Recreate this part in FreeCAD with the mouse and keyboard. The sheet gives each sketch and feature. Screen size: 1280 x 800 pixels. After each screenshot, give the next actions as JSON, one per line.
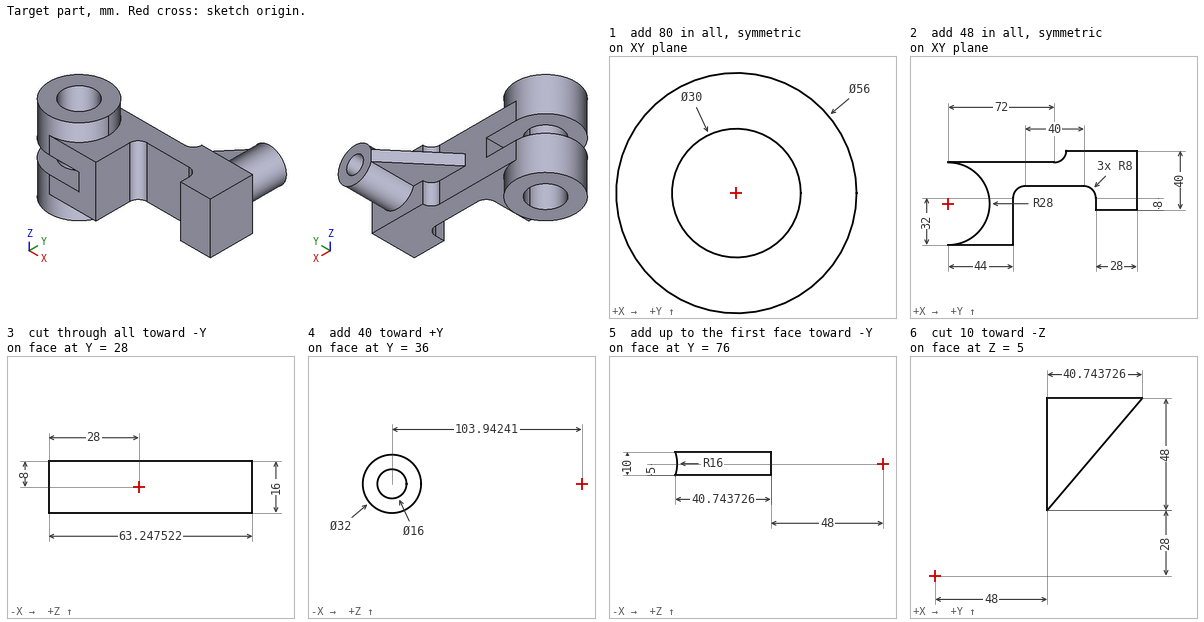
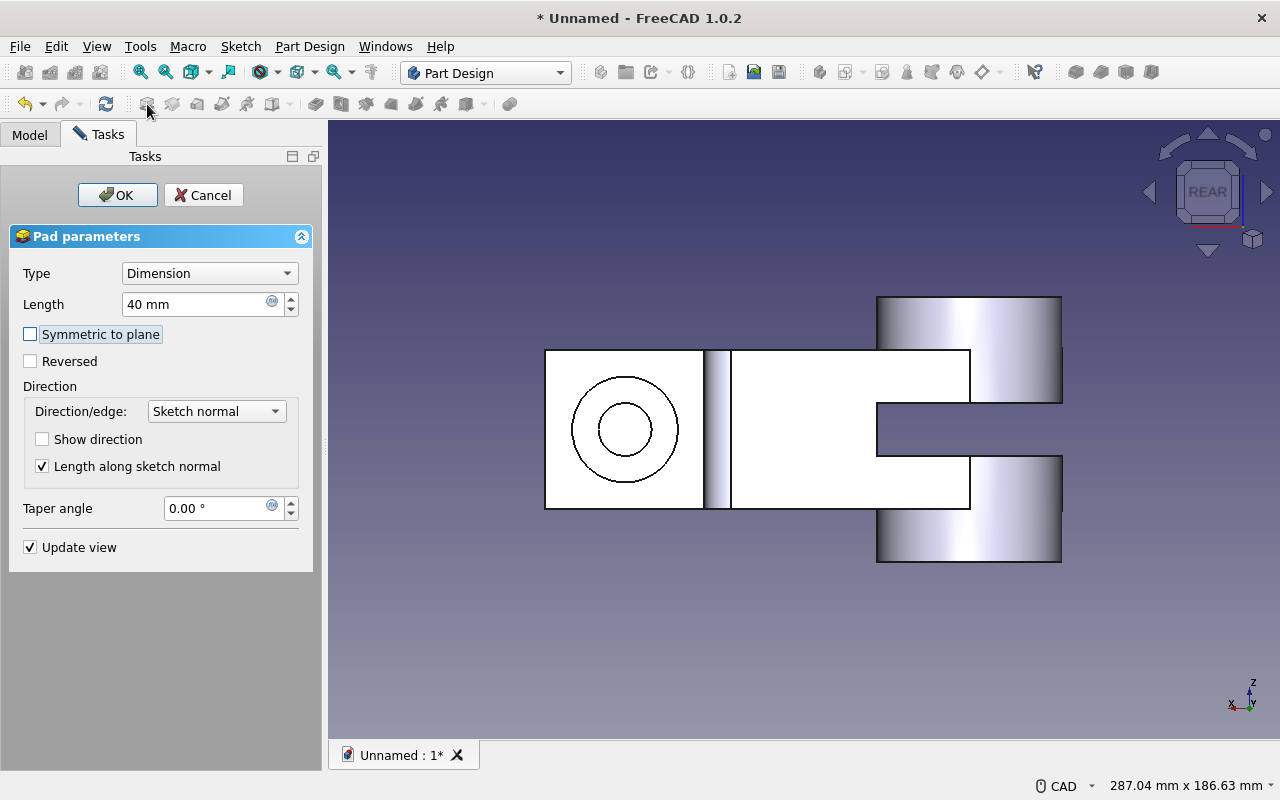
{"action": "left_click", "coordinate": [118, 195]}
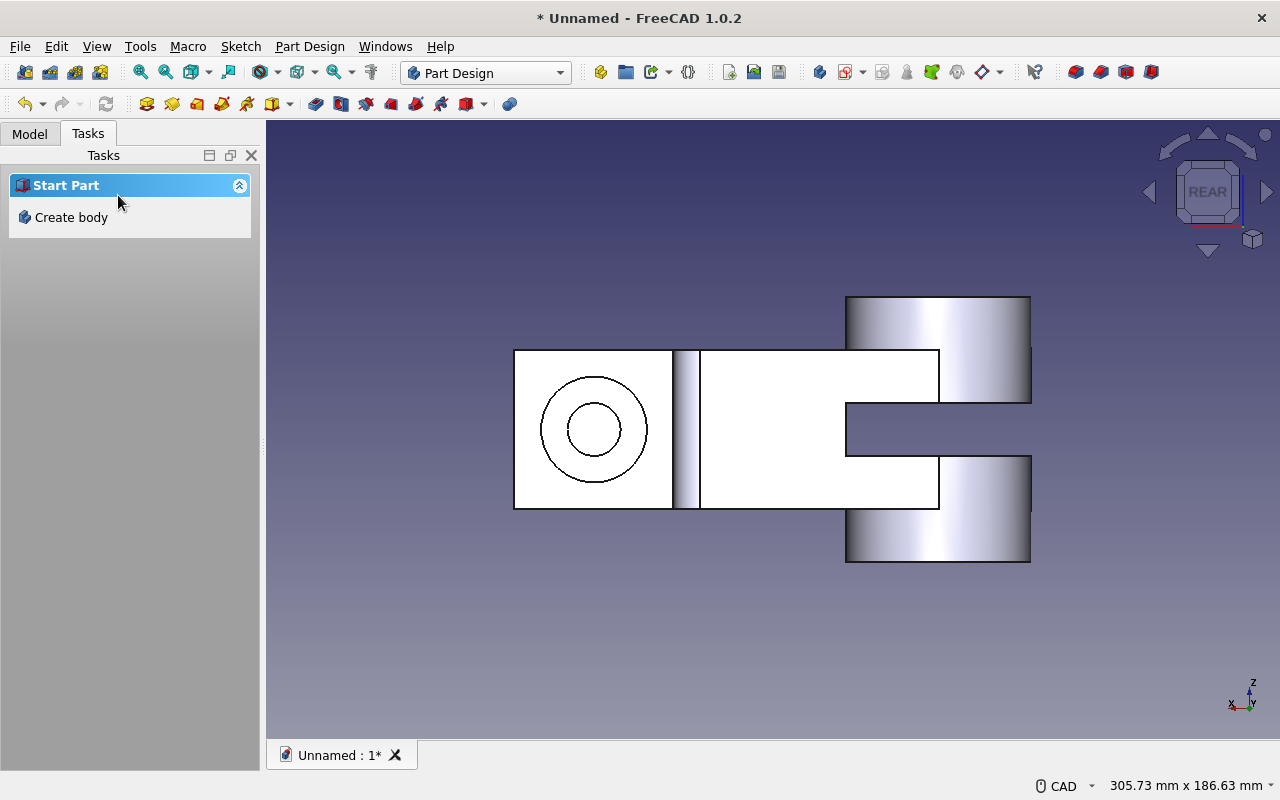
{"action": "left_click", "coordinate": [564, 459]}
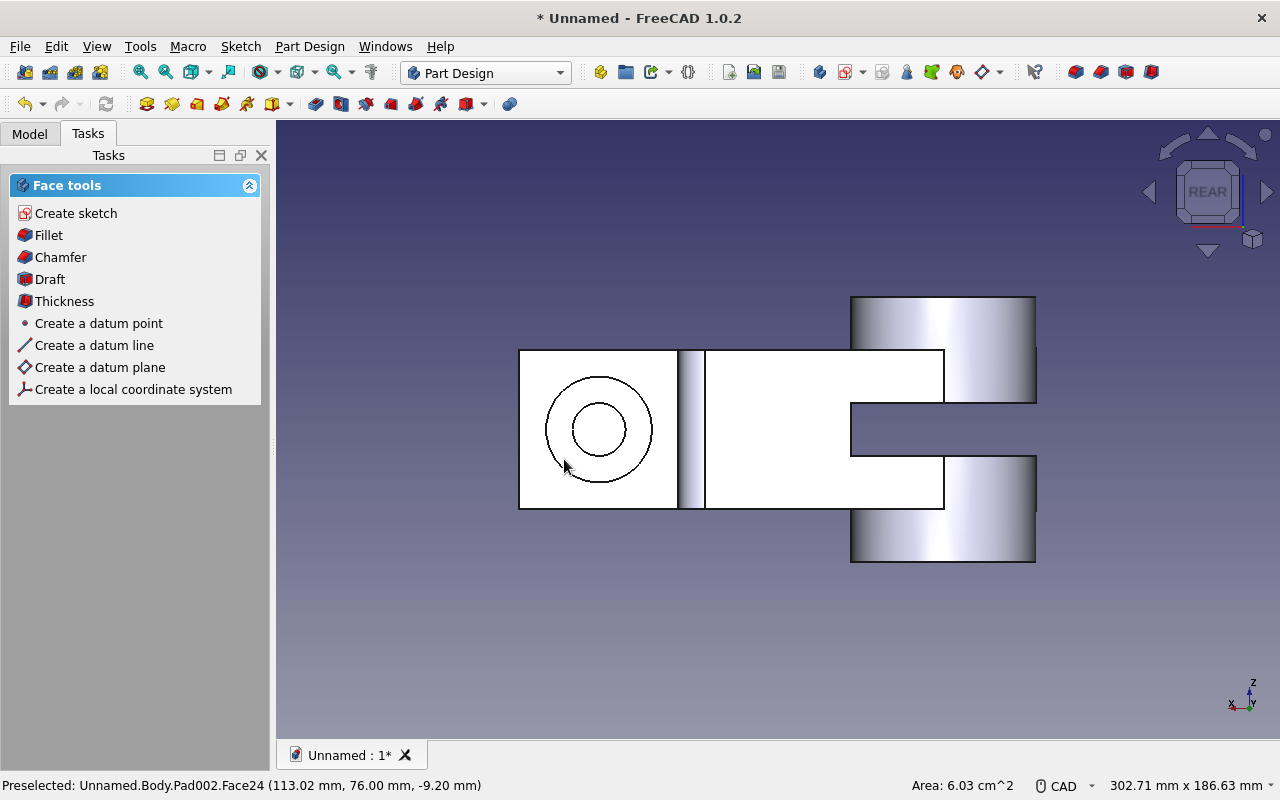
{"action": "left_click", "coordinate": [844, 72]}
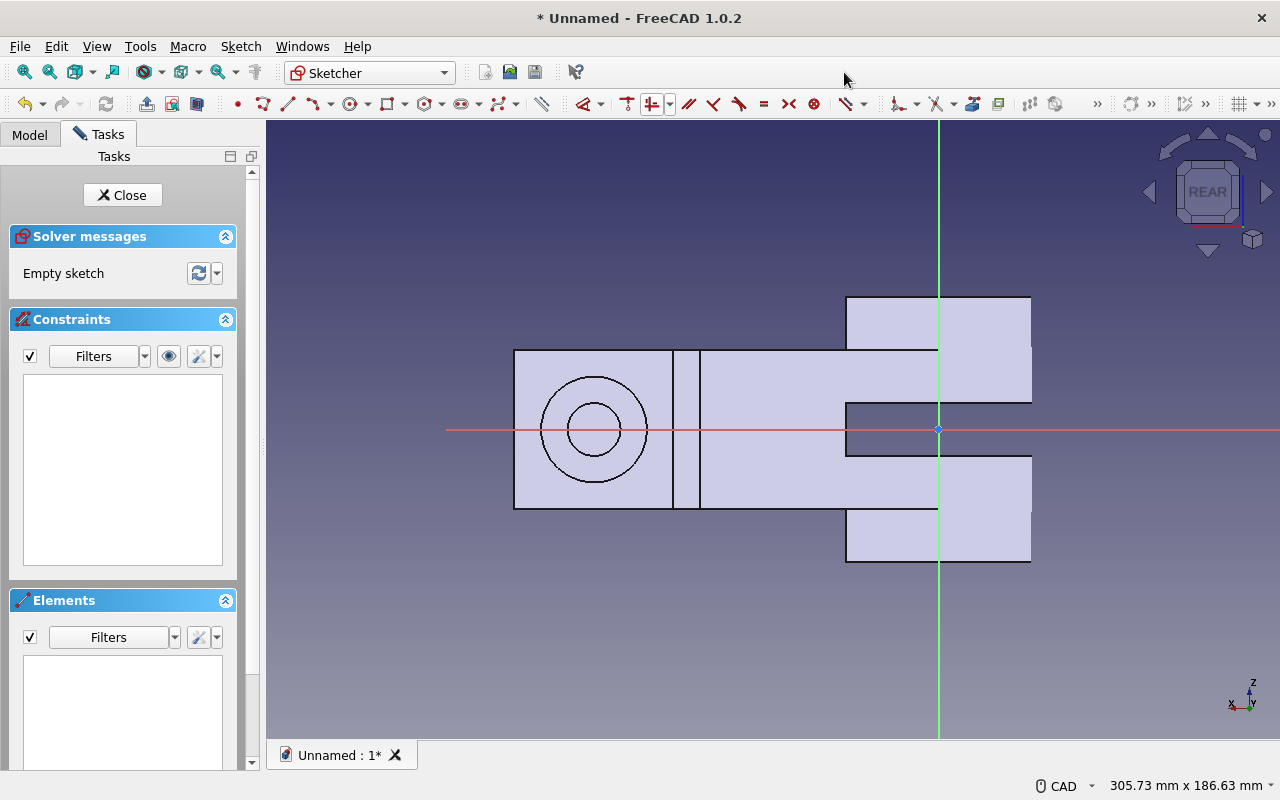
{"action": "scroll", "coordinate": [898, 430], "scroll_direction": "up", "scroll_amount": 3}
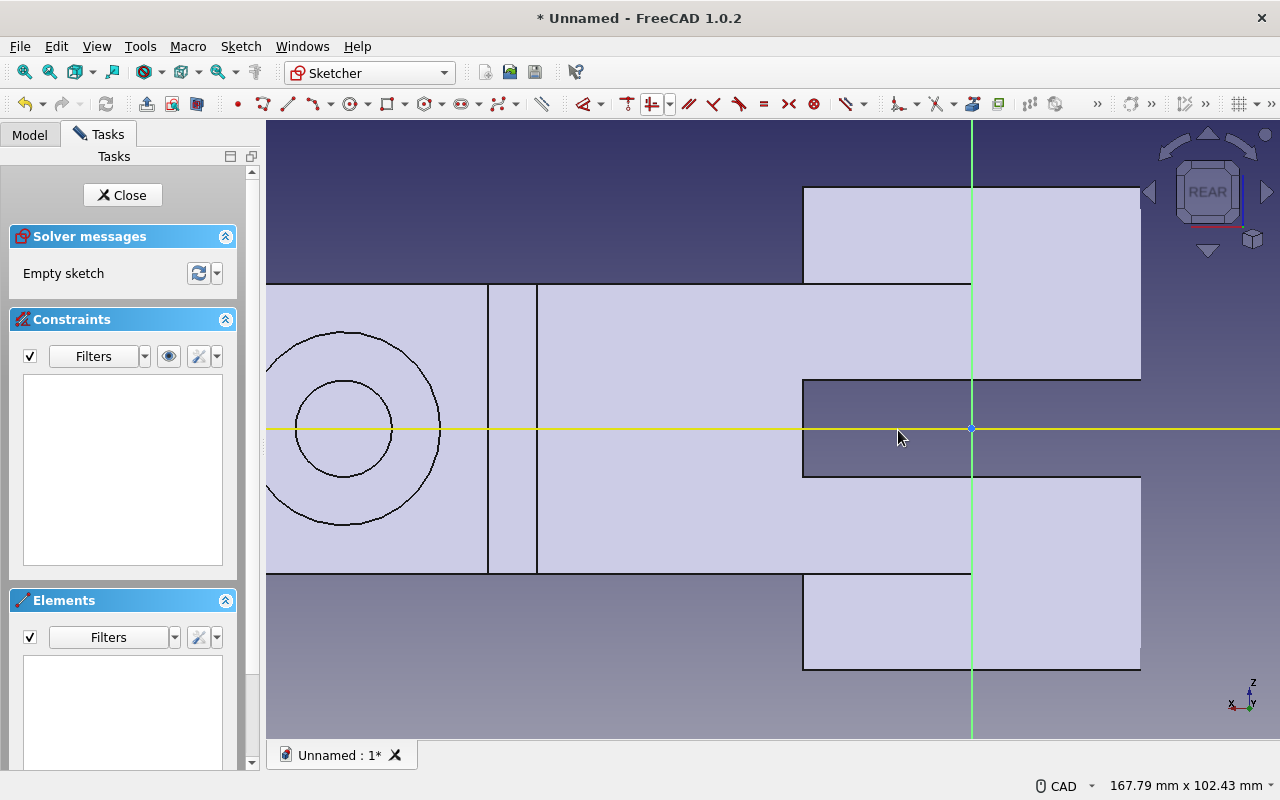
{"action": "left_click", "coordinate": [263, 104]}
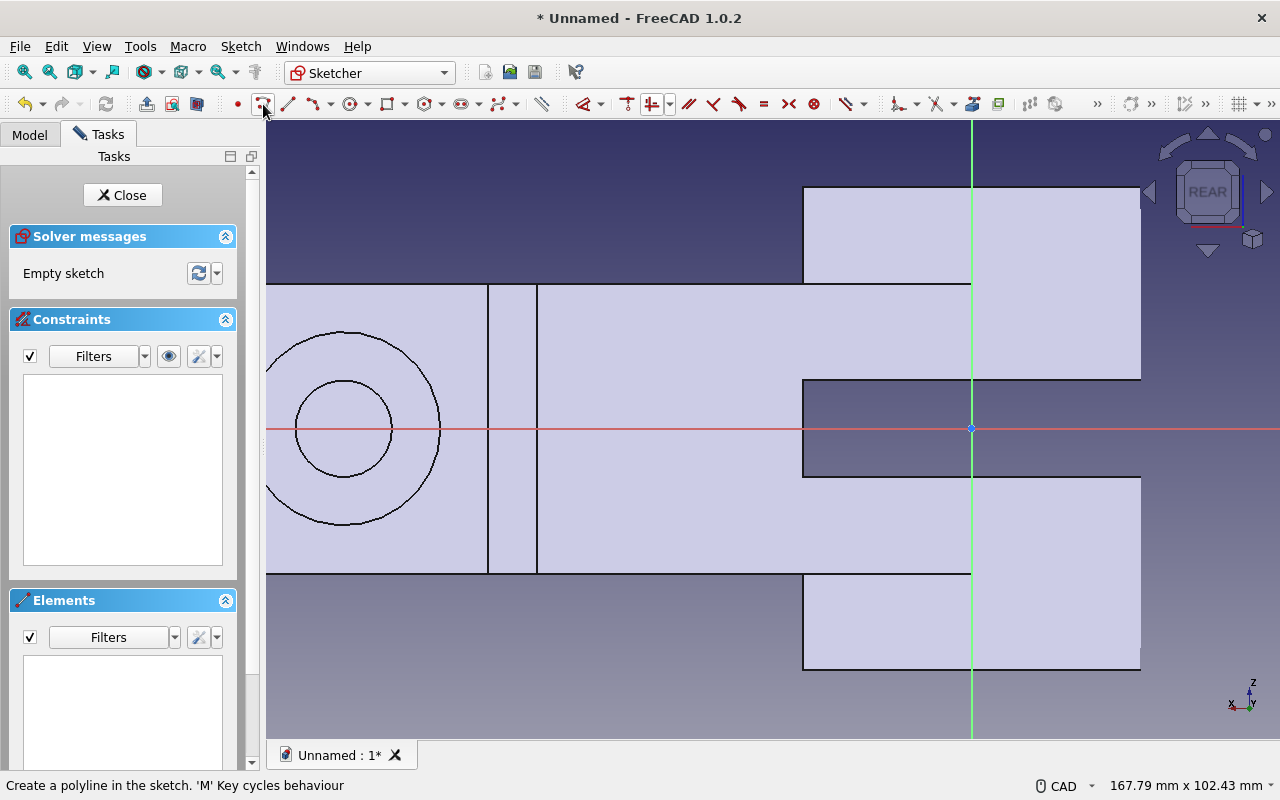
{"action": "left_click", "coordinate": [436, 459]}
{"action": "left_click", "coordinate": [682, 459]}
{"action": "left_click", "coordinate": [682, 398]}
{"action": "left_click", "coordinate": [436, 398]}
{"action": "right_click", "coordinate": [436, 398]}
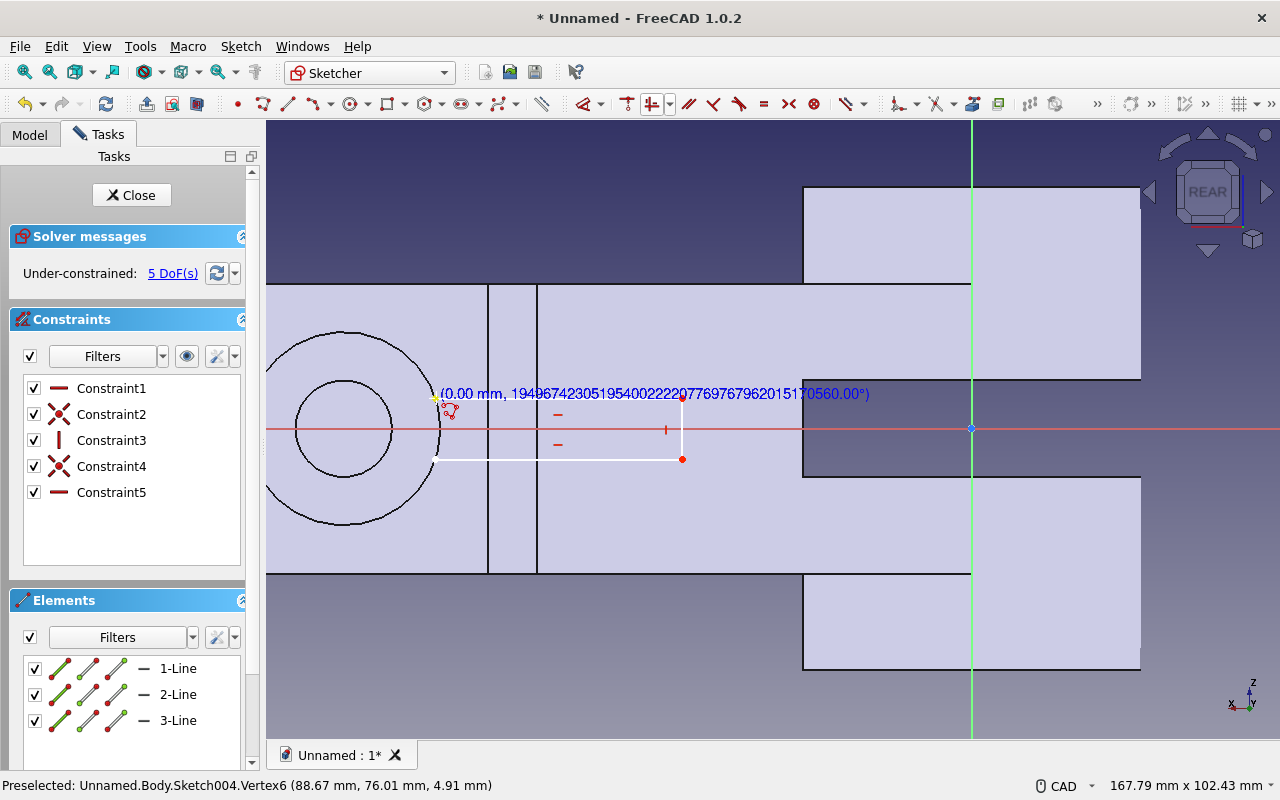
{"action": "left_click", "coordinate": [312, 104]}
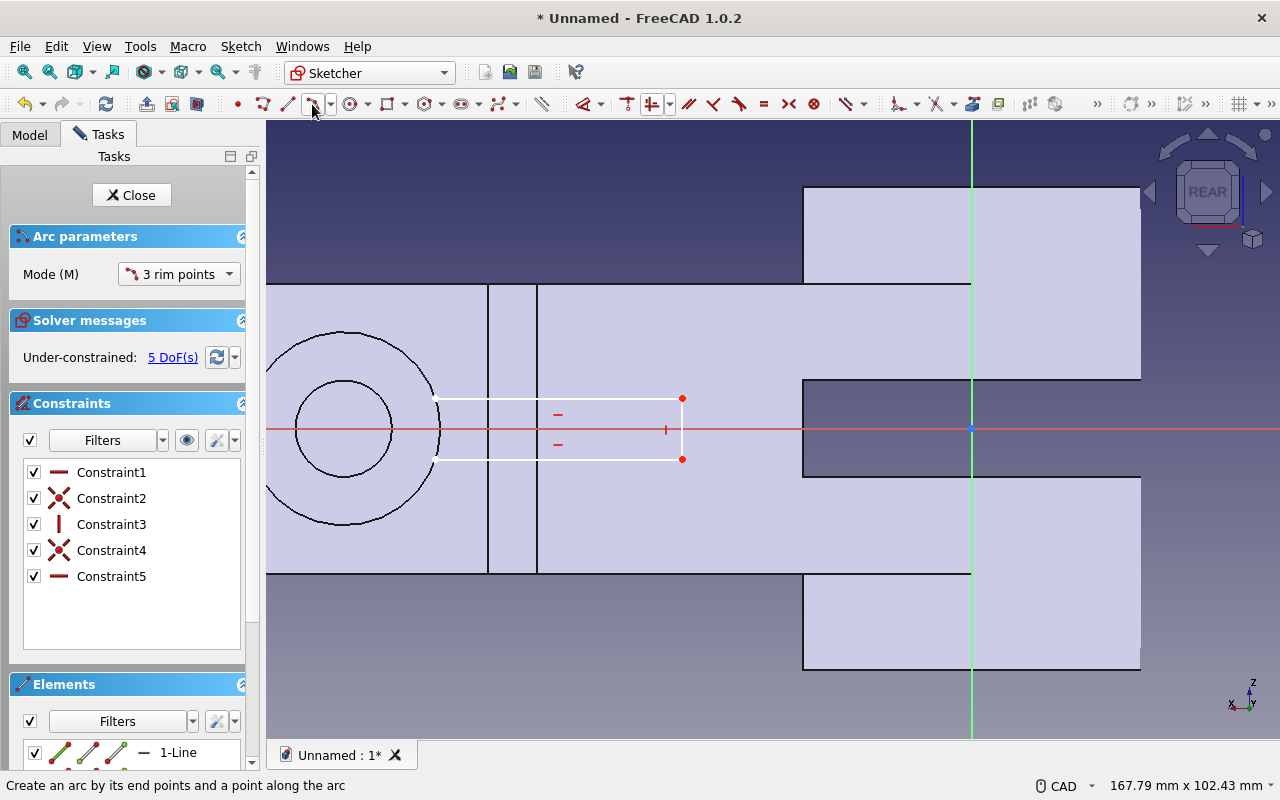
{"action": "left_click", "coordinate": [436, 399]}
{"action": "left_click", "coordinate": [436, 460]}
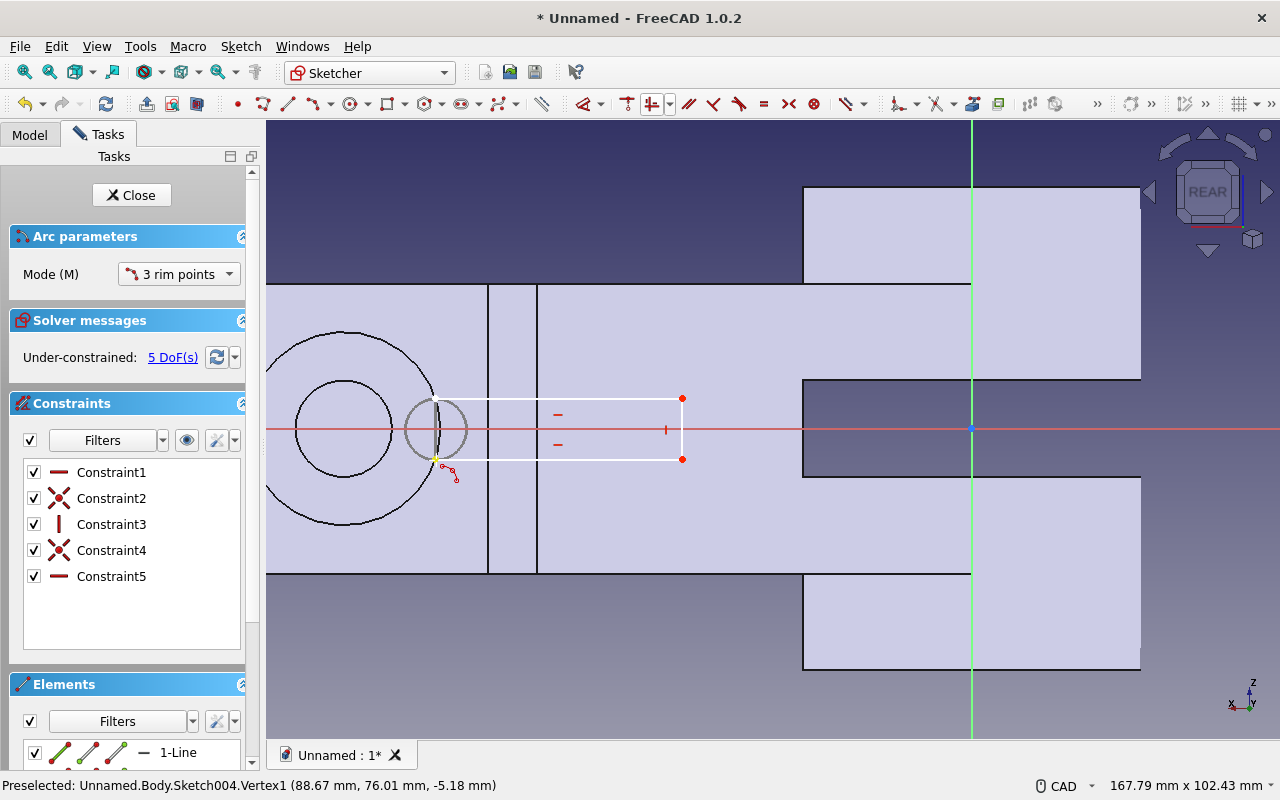
{"action": "scroll", "coordinate": [440, 435], "scroll_direction": "up", "scroll_amount": 7}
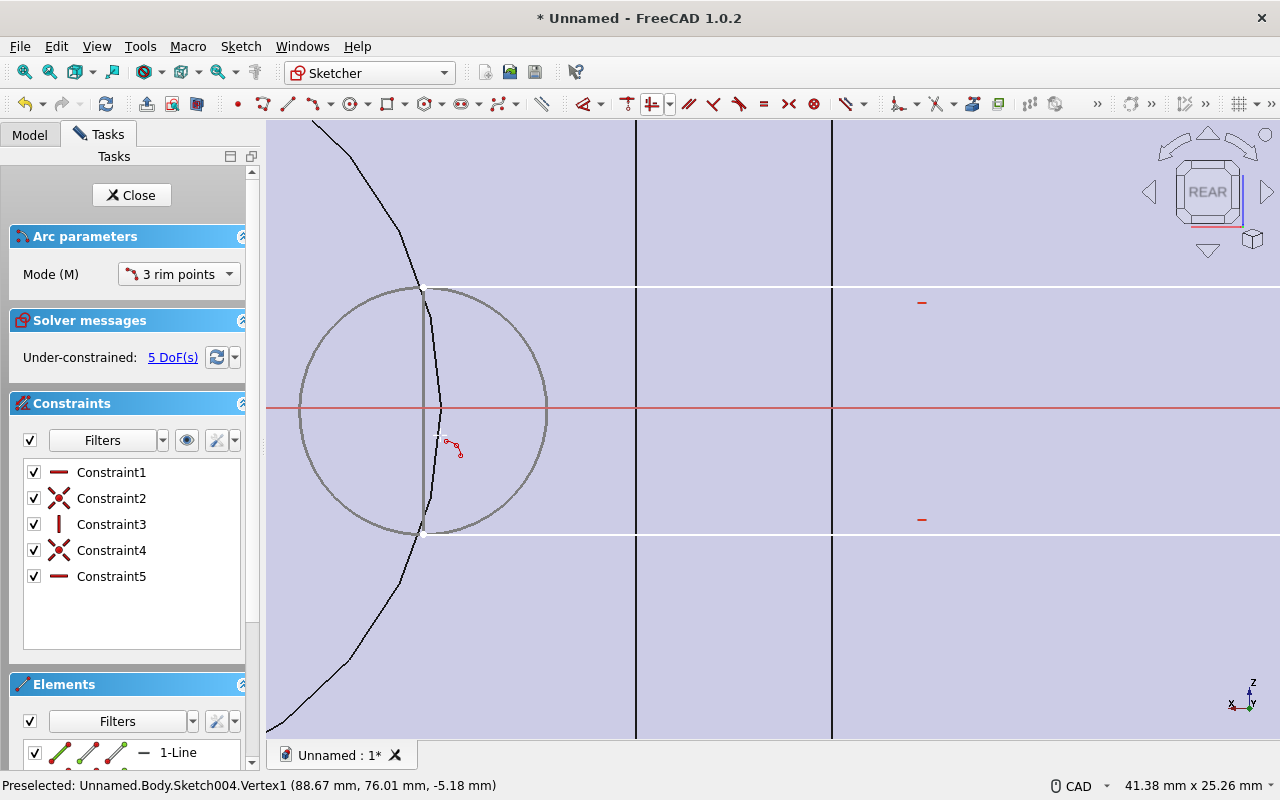
{"action": "left_click", "coordinate": [440, 433]}
{"action": "key", "text": "Escape"}